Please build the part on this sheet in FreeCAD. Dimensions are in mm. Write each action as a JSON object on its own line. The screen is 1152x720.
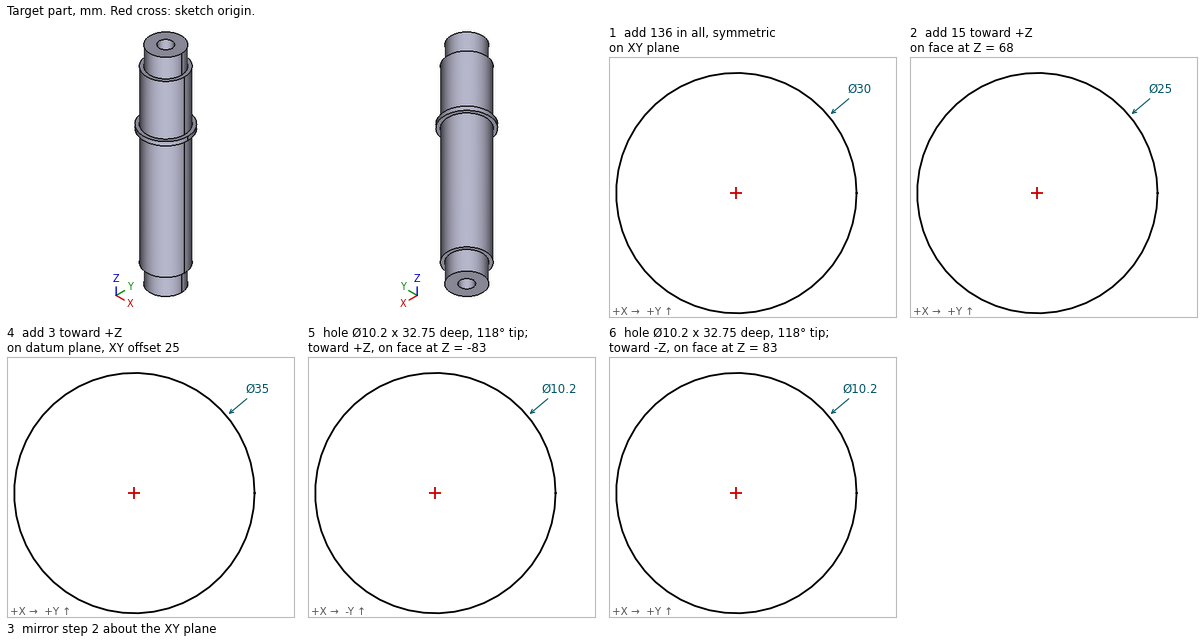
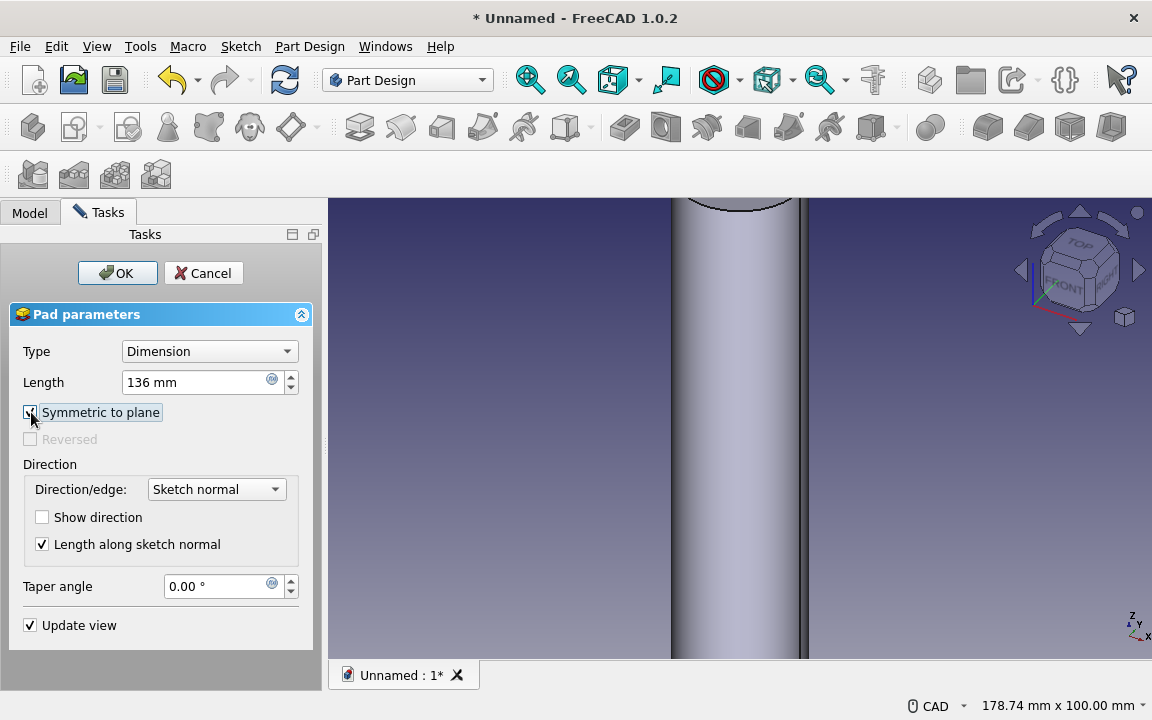
{"action": "left_click", "coordinate": [118, 273]}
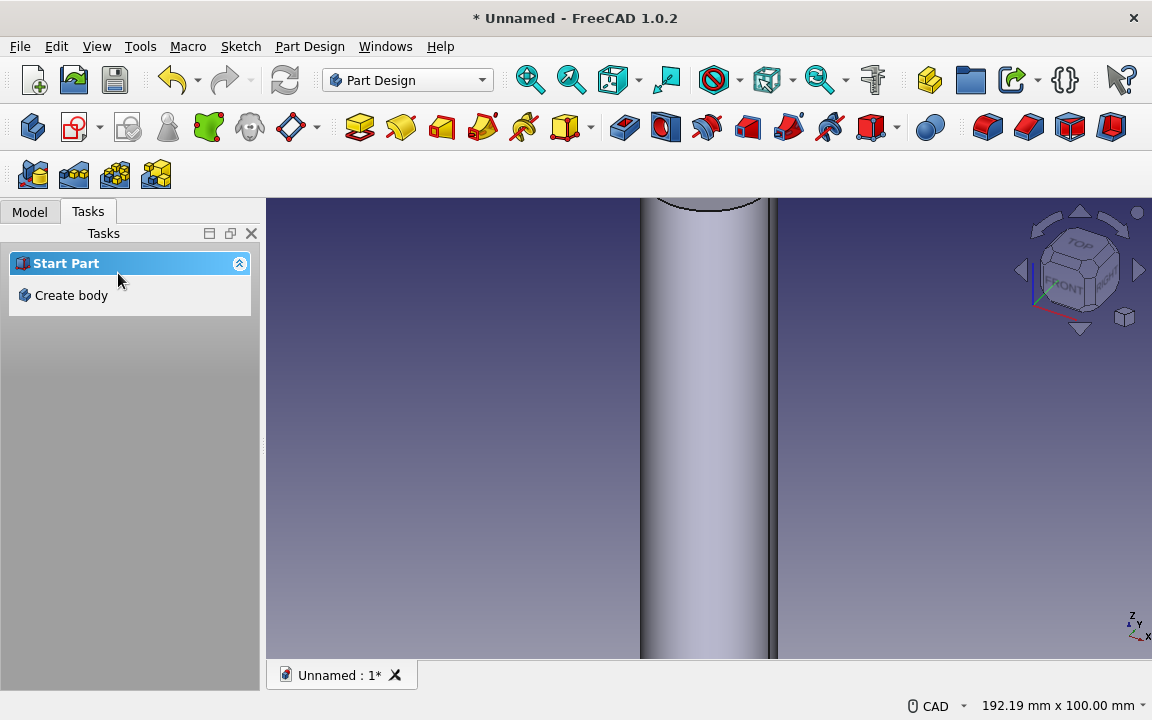
{"action": "left_click", "coordinate": [531, 80]}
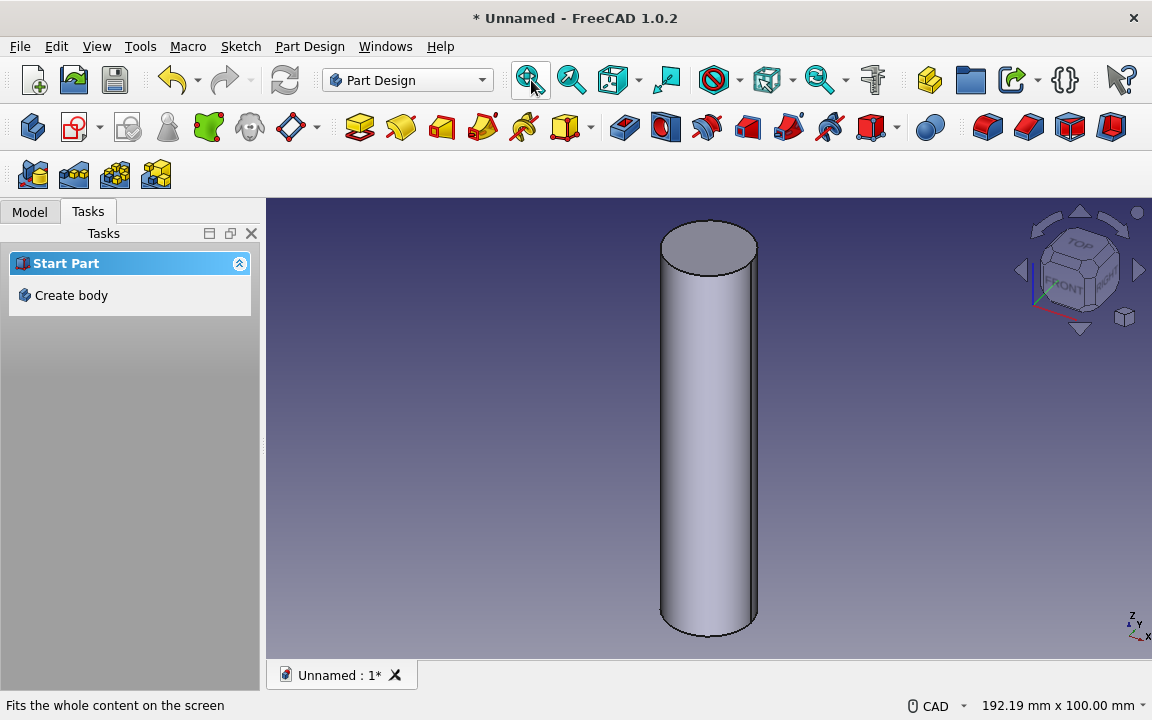
{"action": "left_click", "coordinate": [709, 247]}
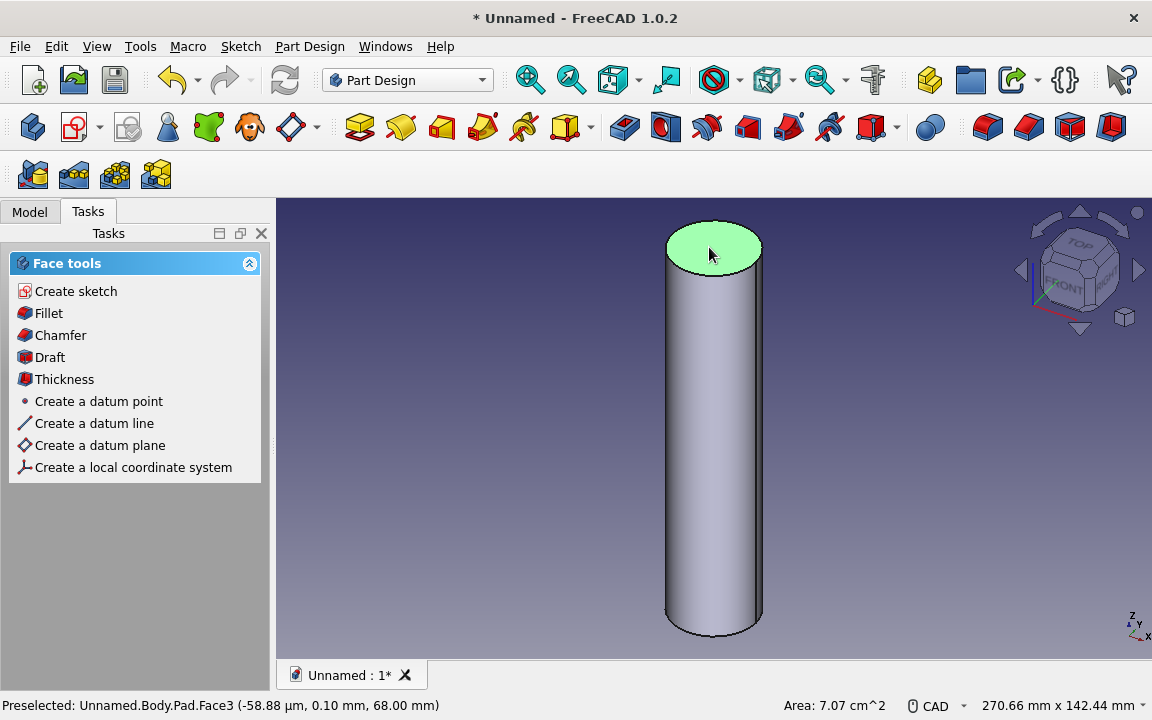
{"action": "left_click", "coordinate": [74, 128]}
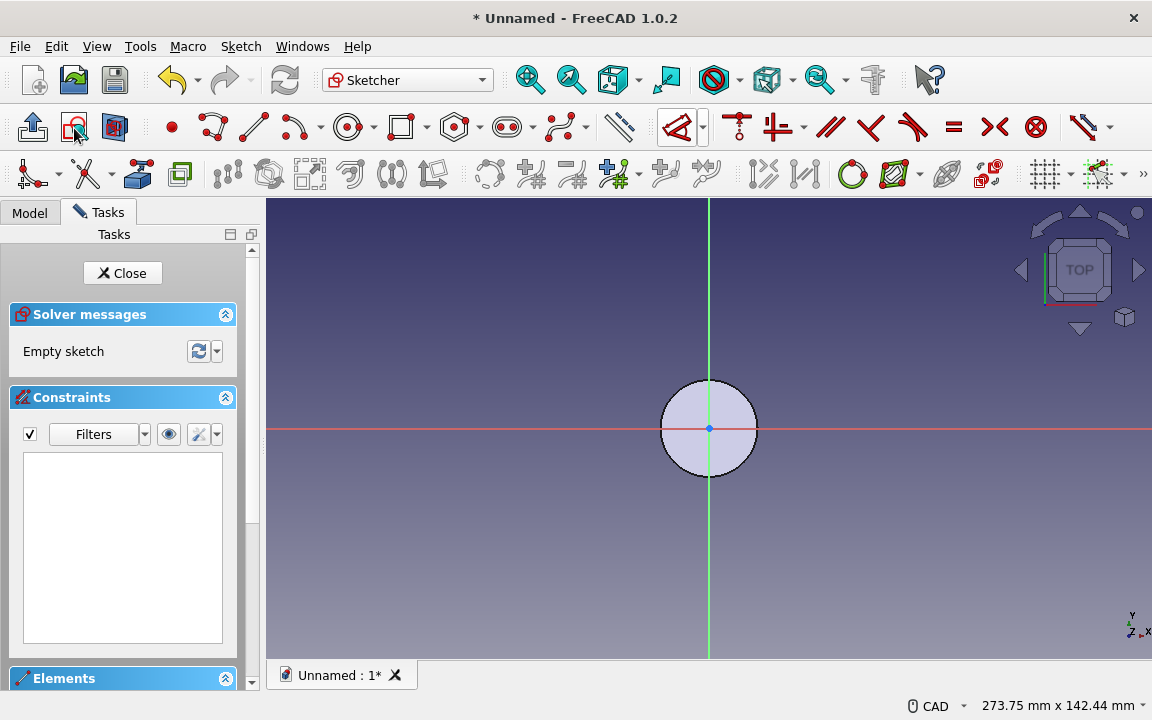
{"action": "scroll", "coordinate": [739, 428], "scroll_direction": "up", "scroll_amount": 6}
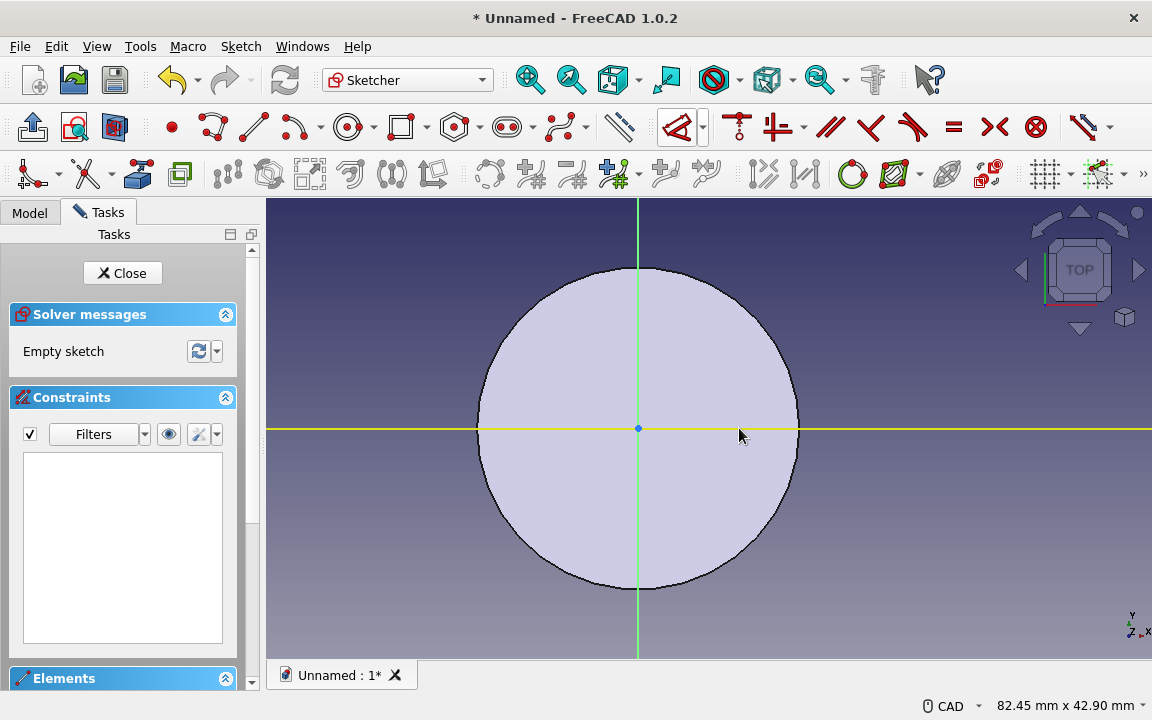
{"action": "left_click", "coordinate": [348, 128]}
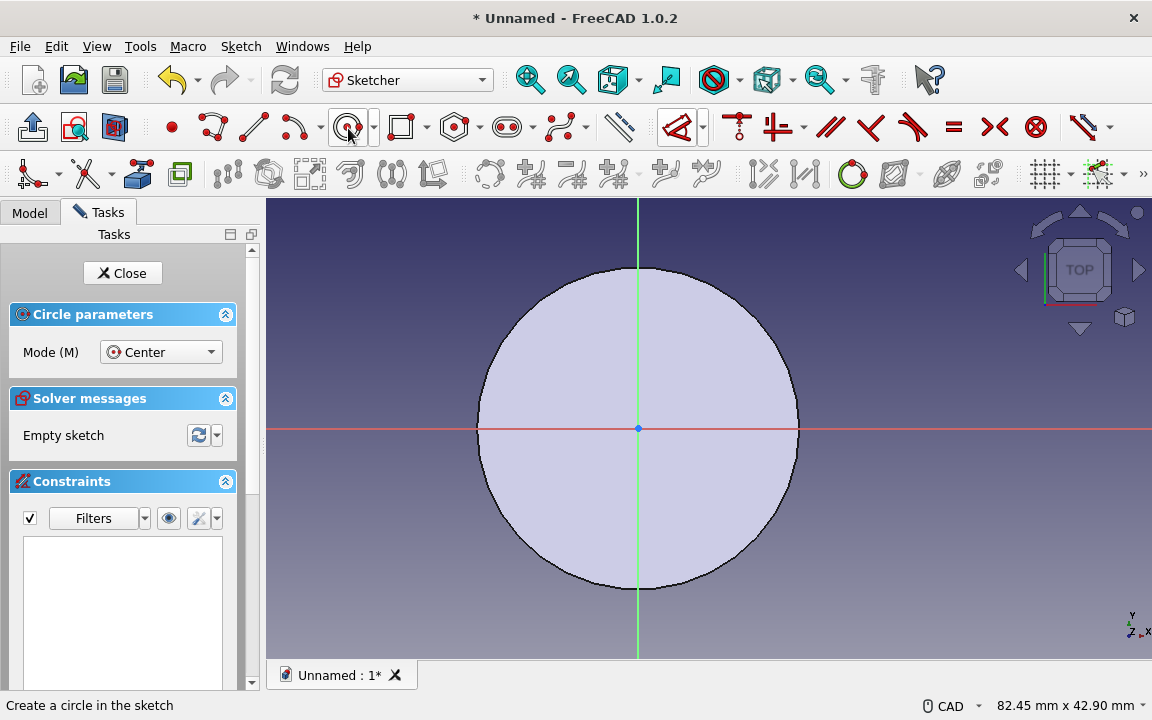
{"action": "left_click", "coordinate": [638, 428]}
{"action": "mouse_move", "coordinate": [733, 334]}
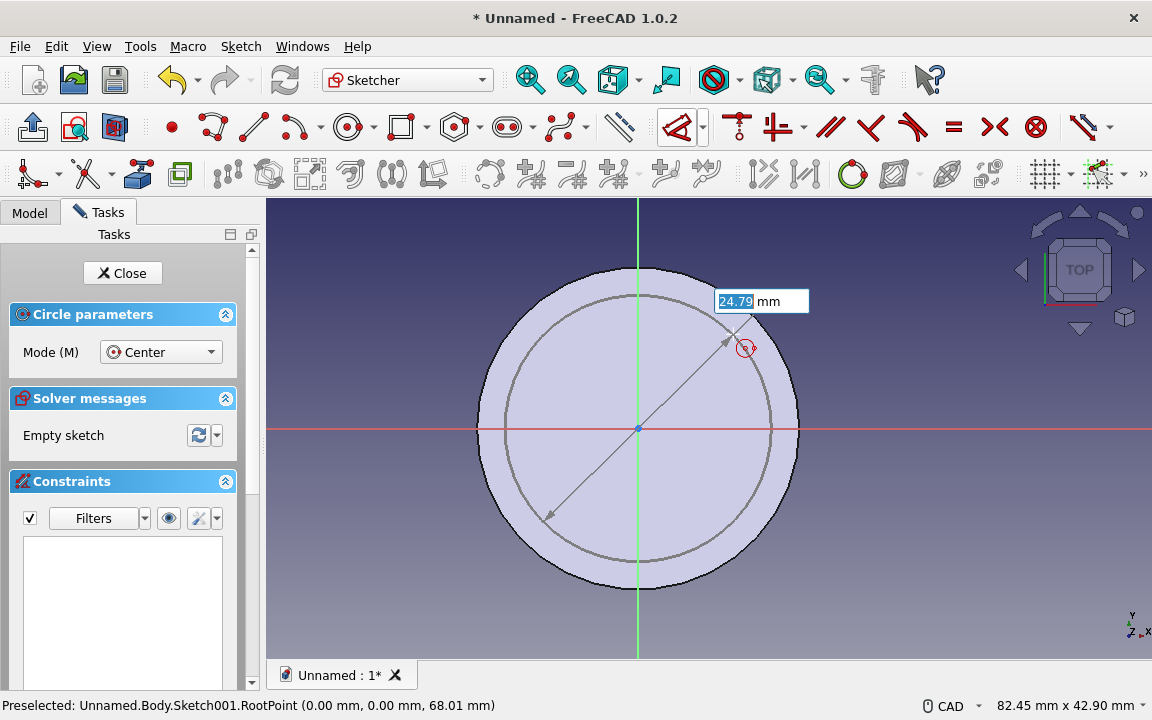
{"action": "type", "text": "25"}
{"action": "key", "text": "Return"}
{"action": "key", "text": "Escape"}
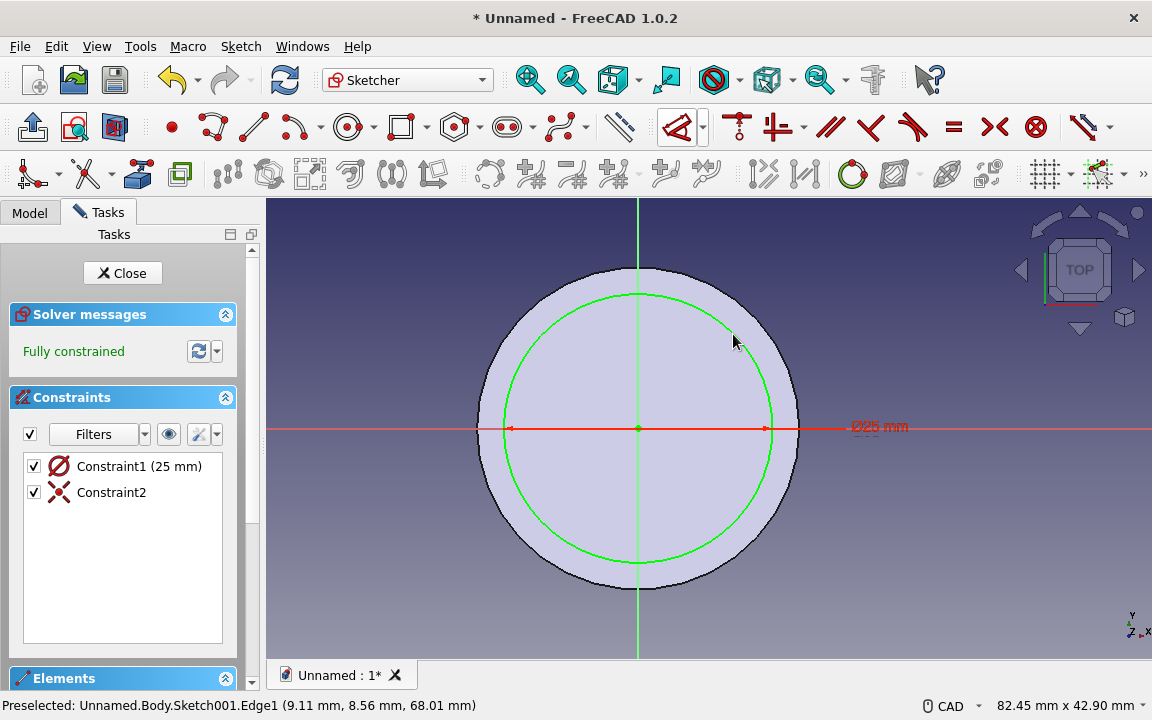
{"action": "left_click", "coordinate": [123, 273]}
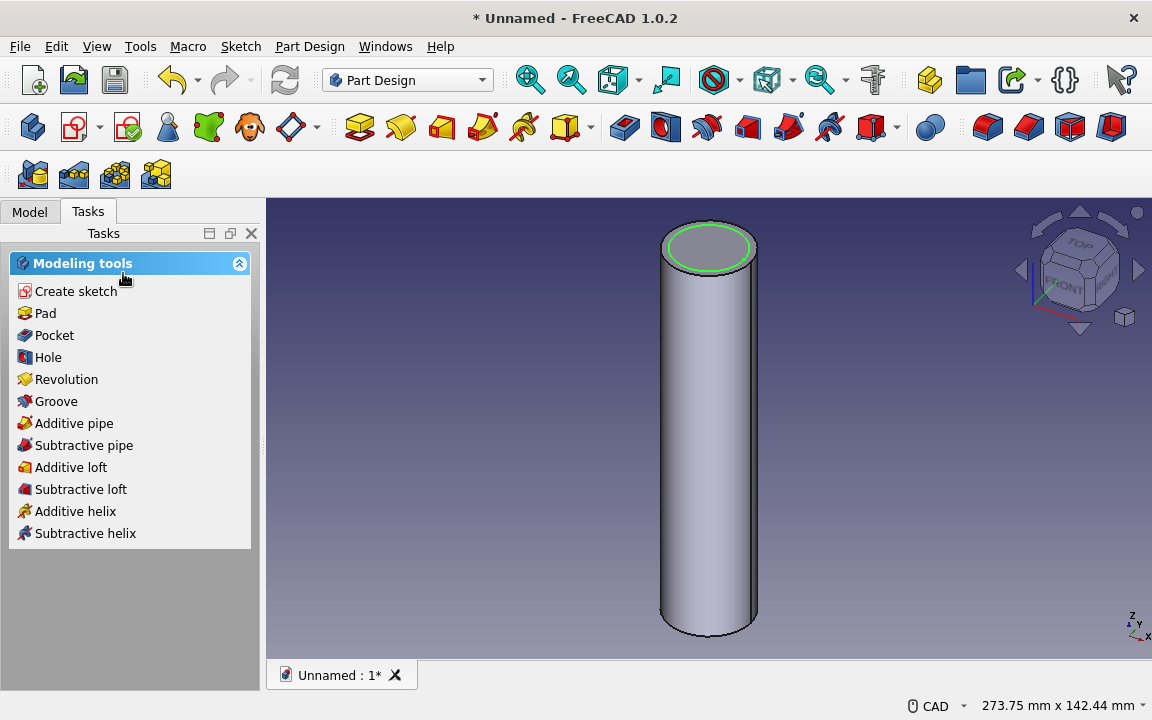
{"action": "left_click", "coordinate": [360, 128]}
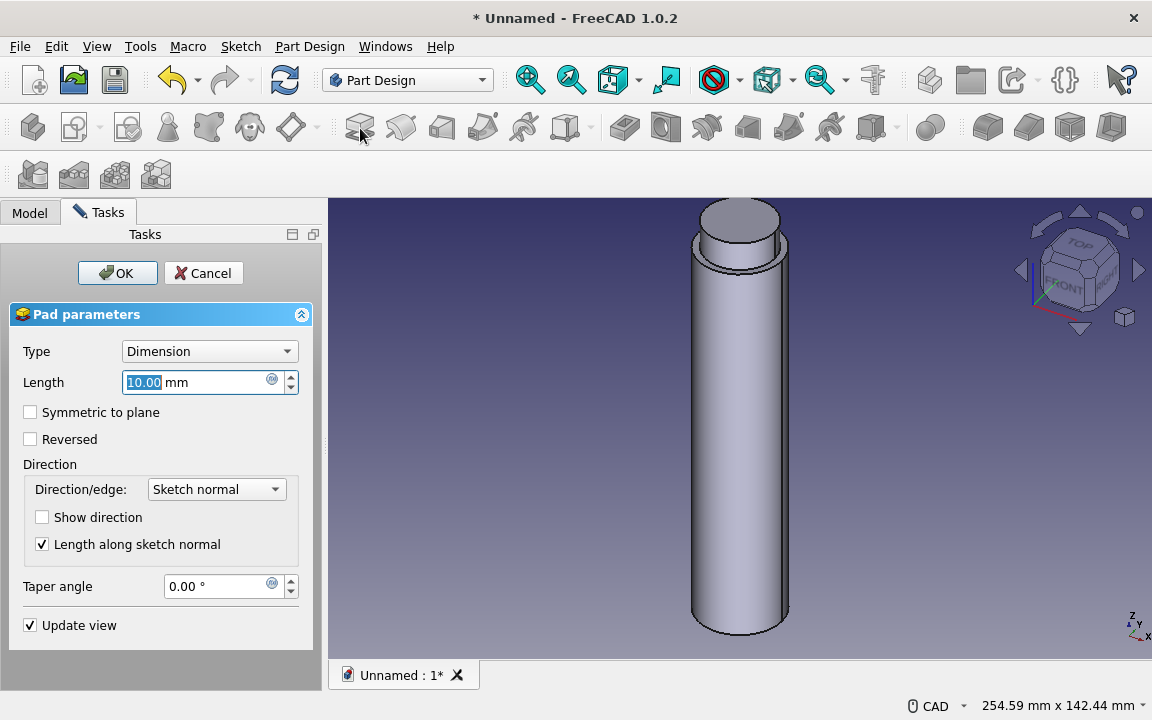
{"action": "type", "text": "15"}
{"action": "key", "text": "Tab"}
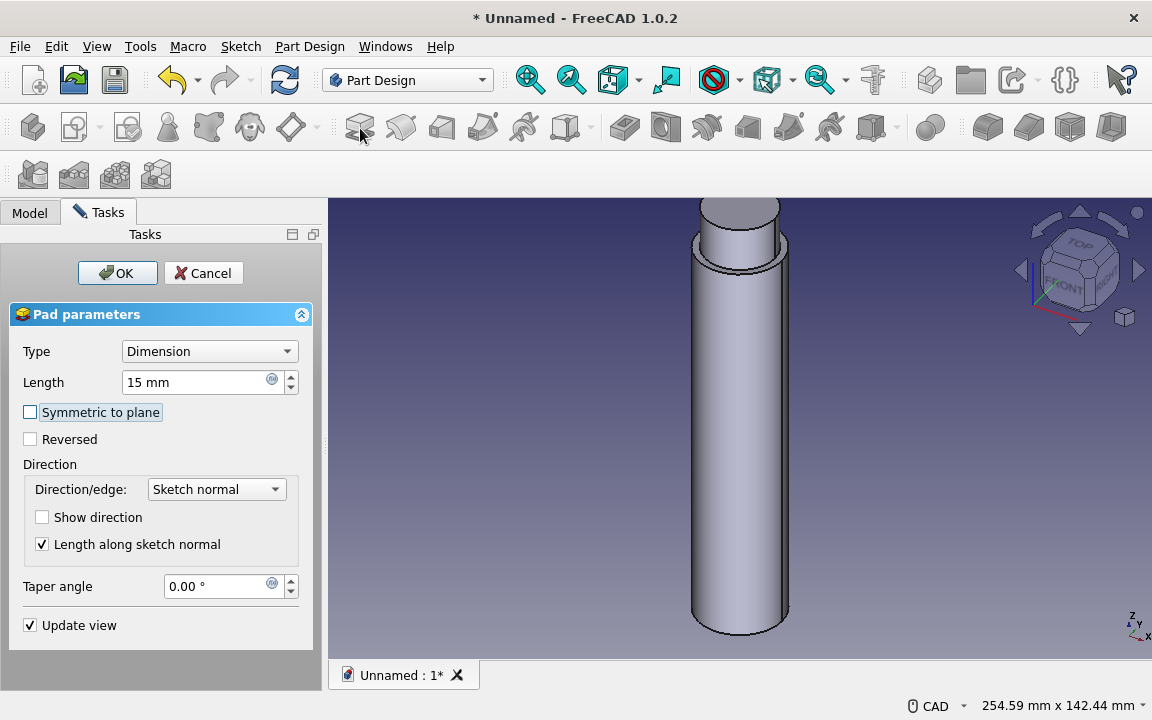
{"action": "left_click", "coordinate": [118, 273]}